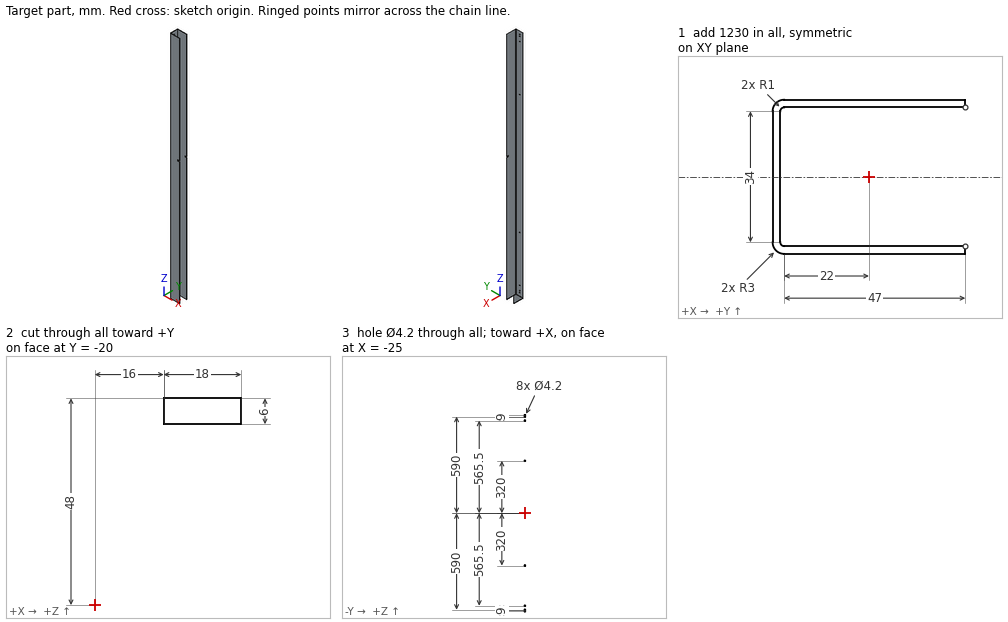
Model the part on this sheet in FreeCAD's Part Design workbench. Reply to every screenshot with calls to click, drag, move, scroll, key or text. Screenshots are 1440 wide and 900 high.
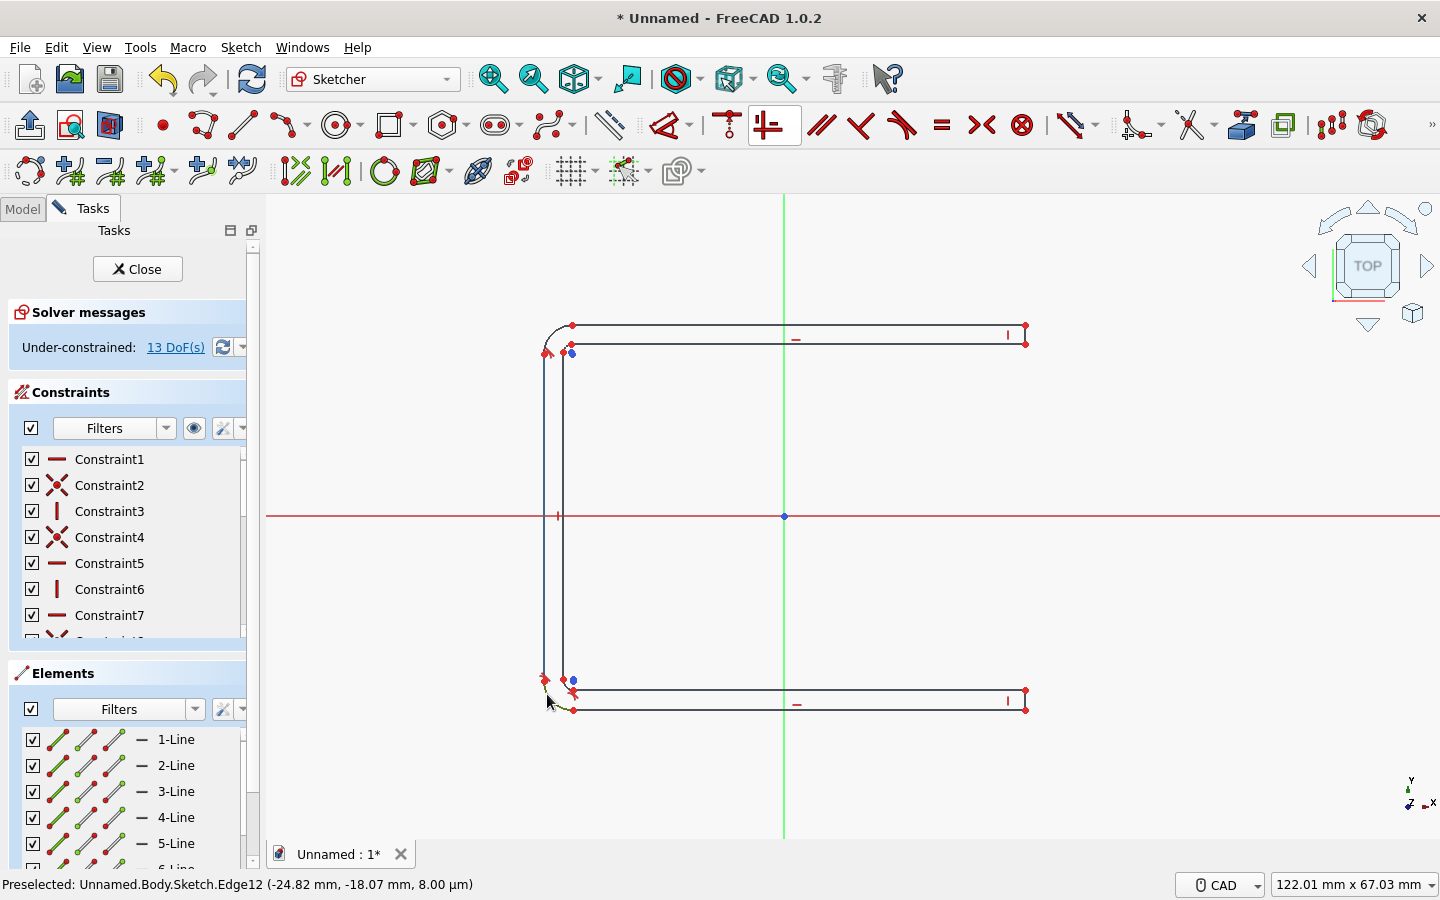
key(t)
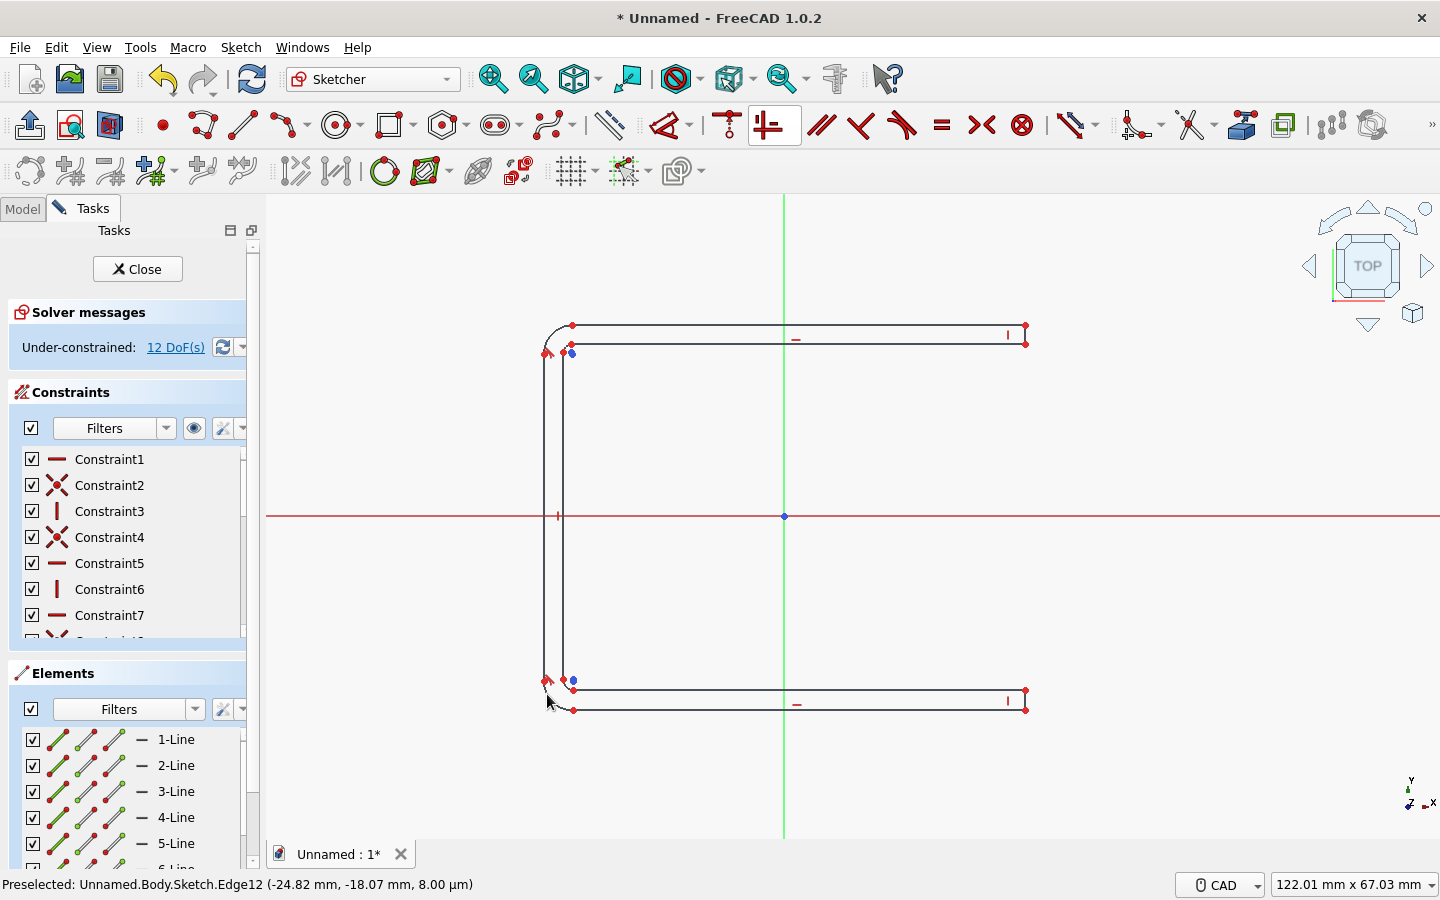
scroll(566, 347, up, 4)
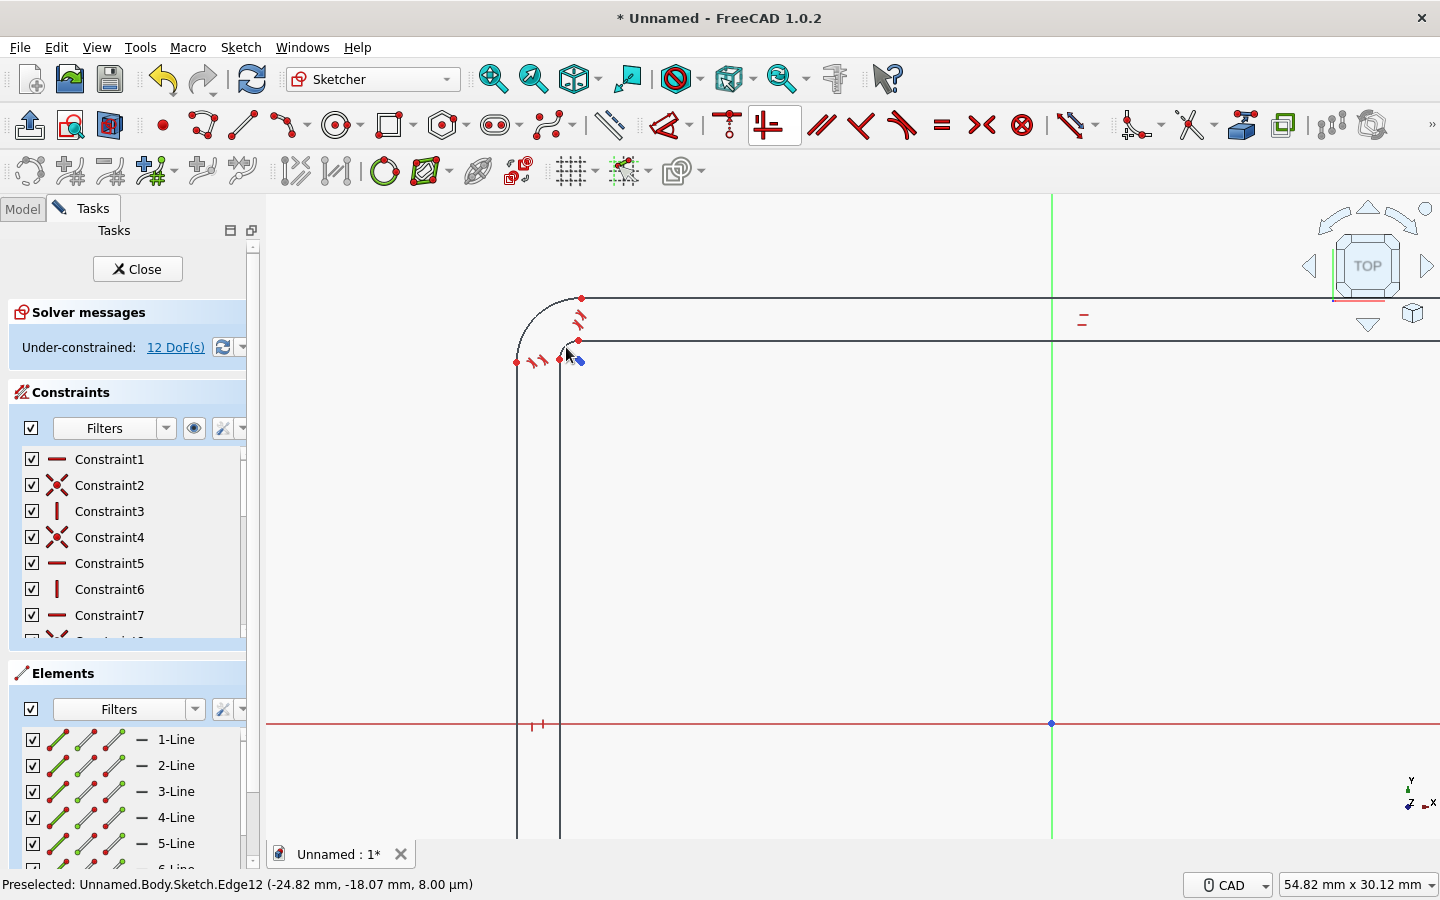
click(565, 346)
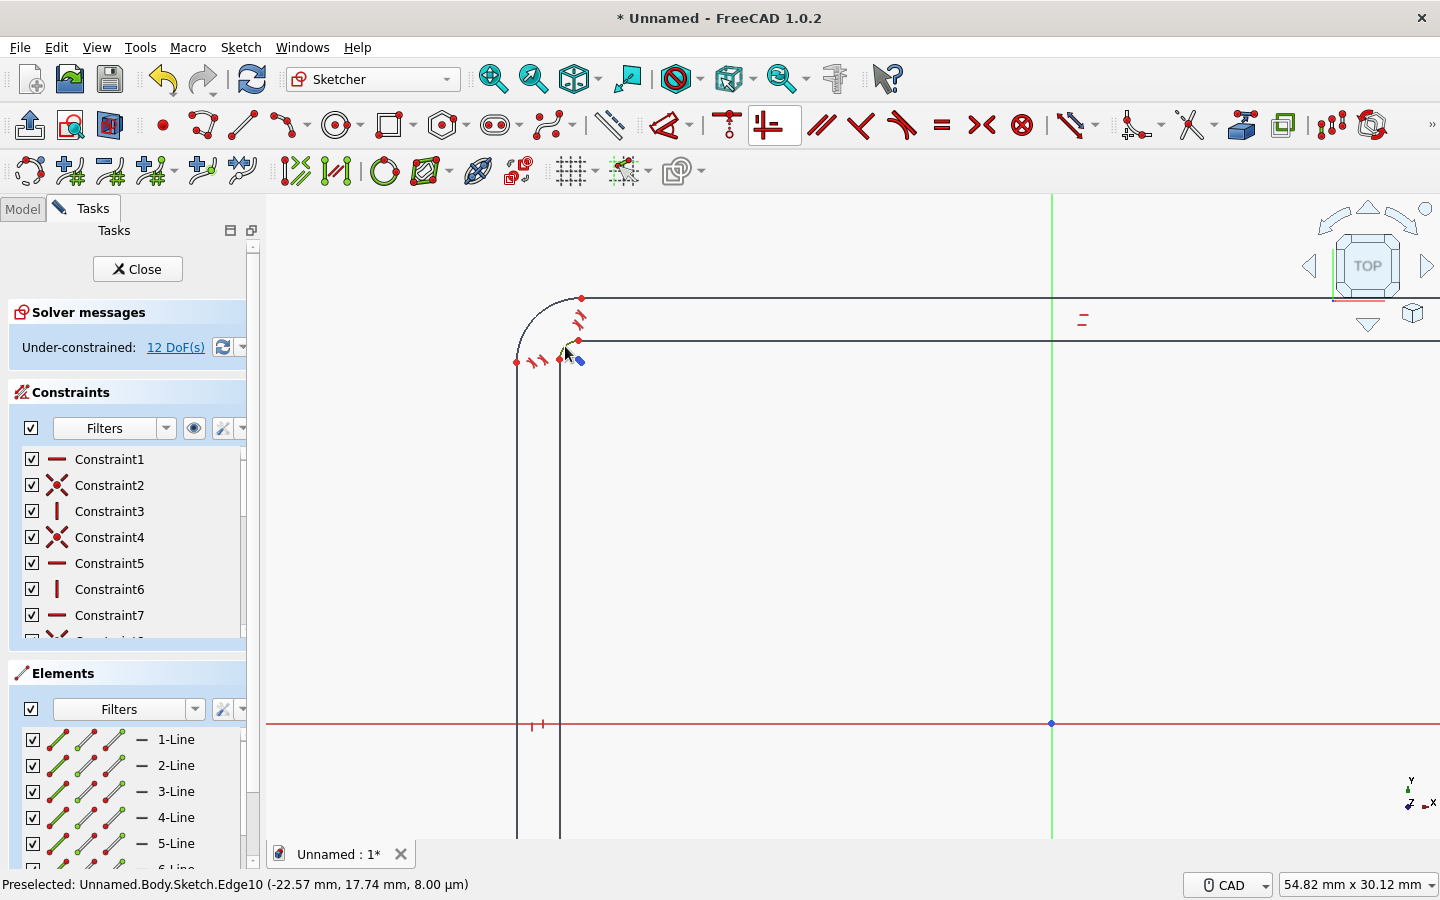
click(552, 305)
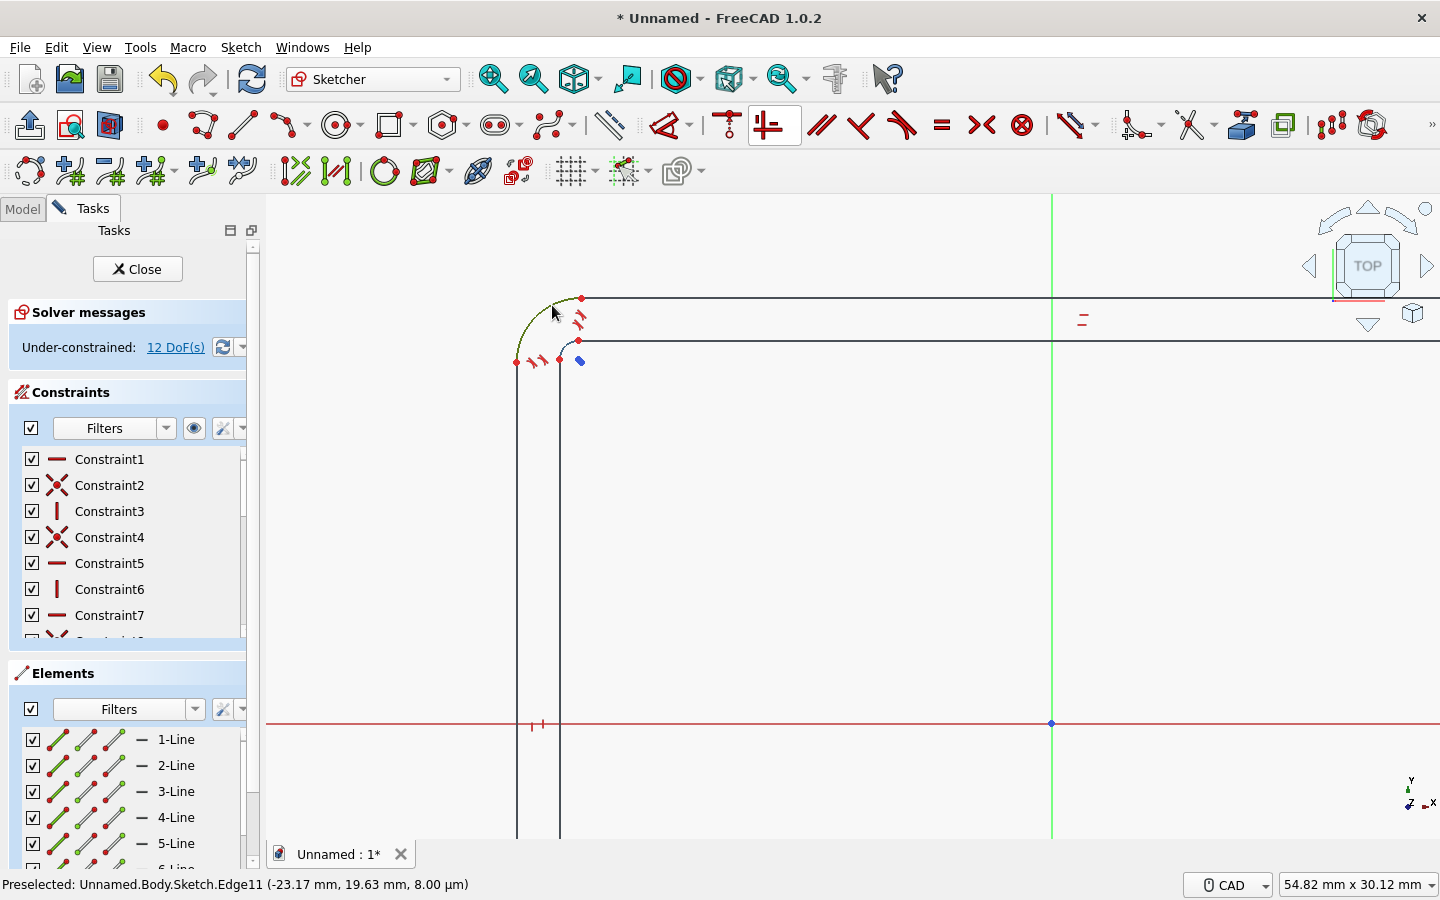
click(728, 126)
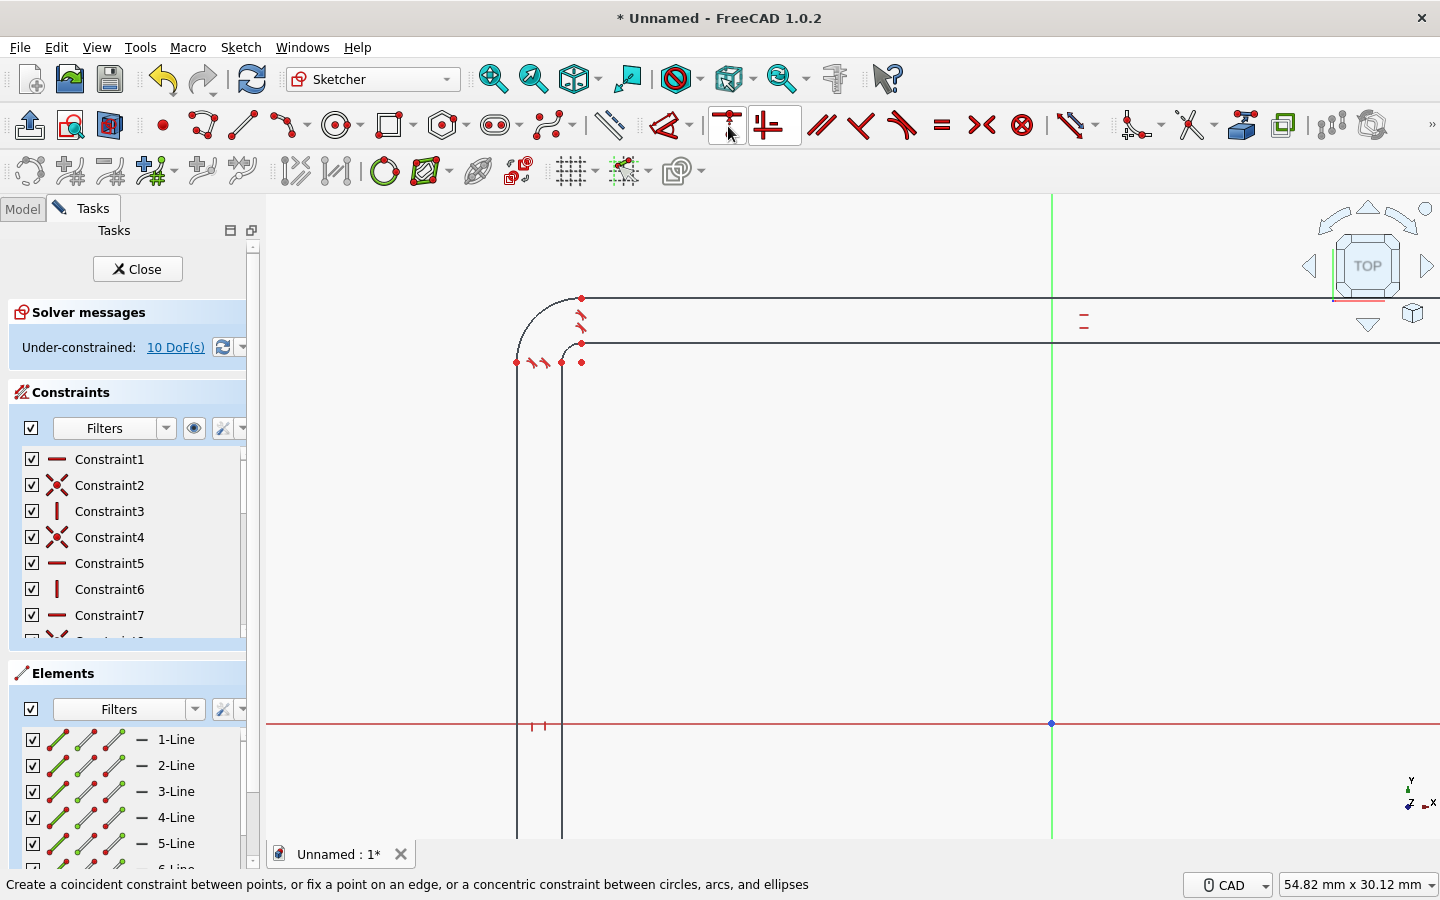
scroll(566, 347, down, 4)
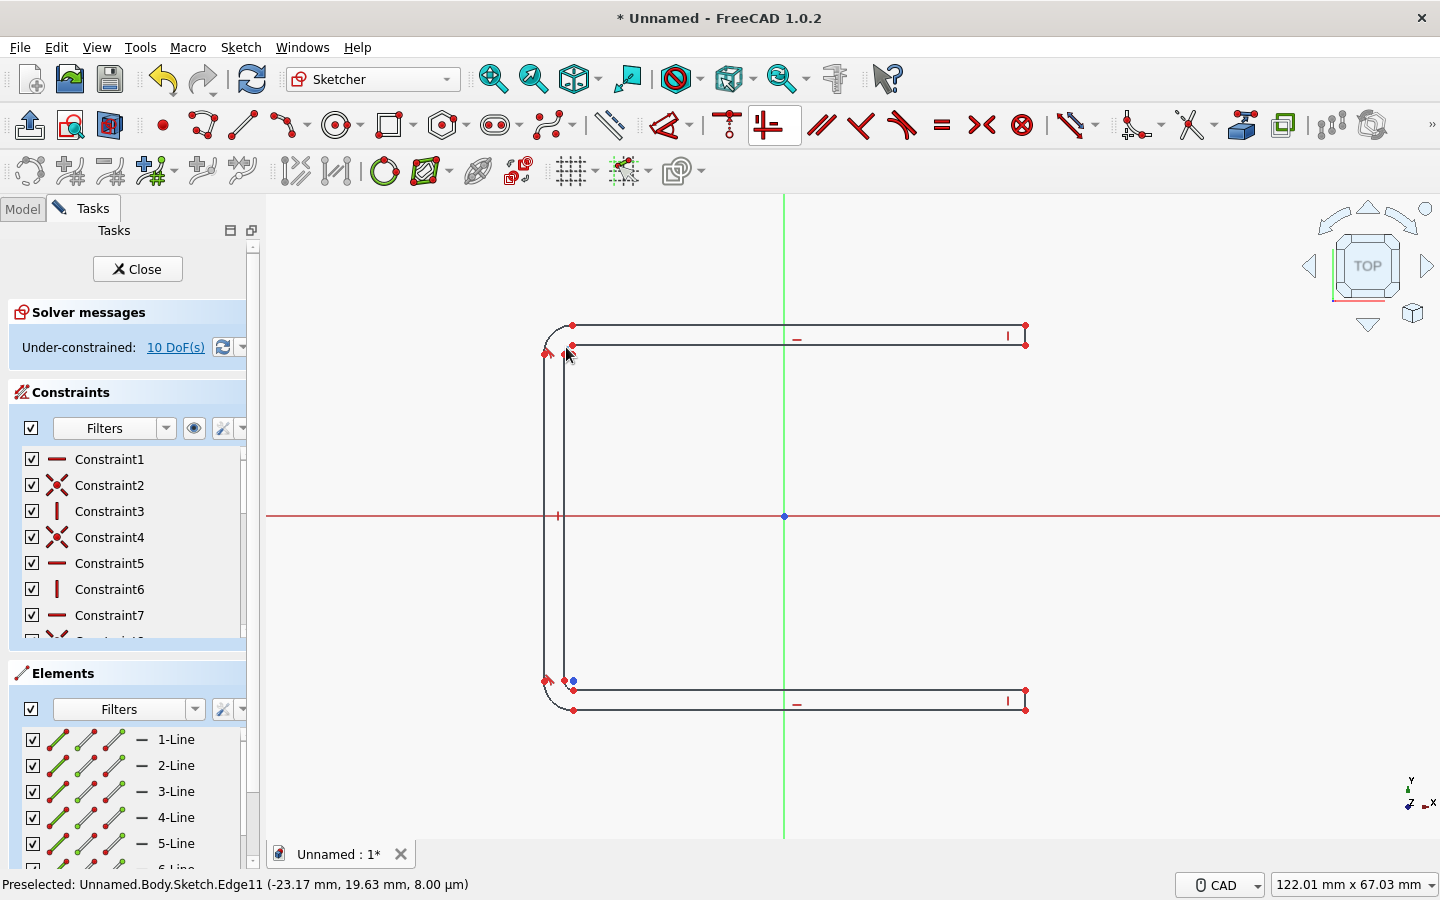
scroll(565, 685, up, 6)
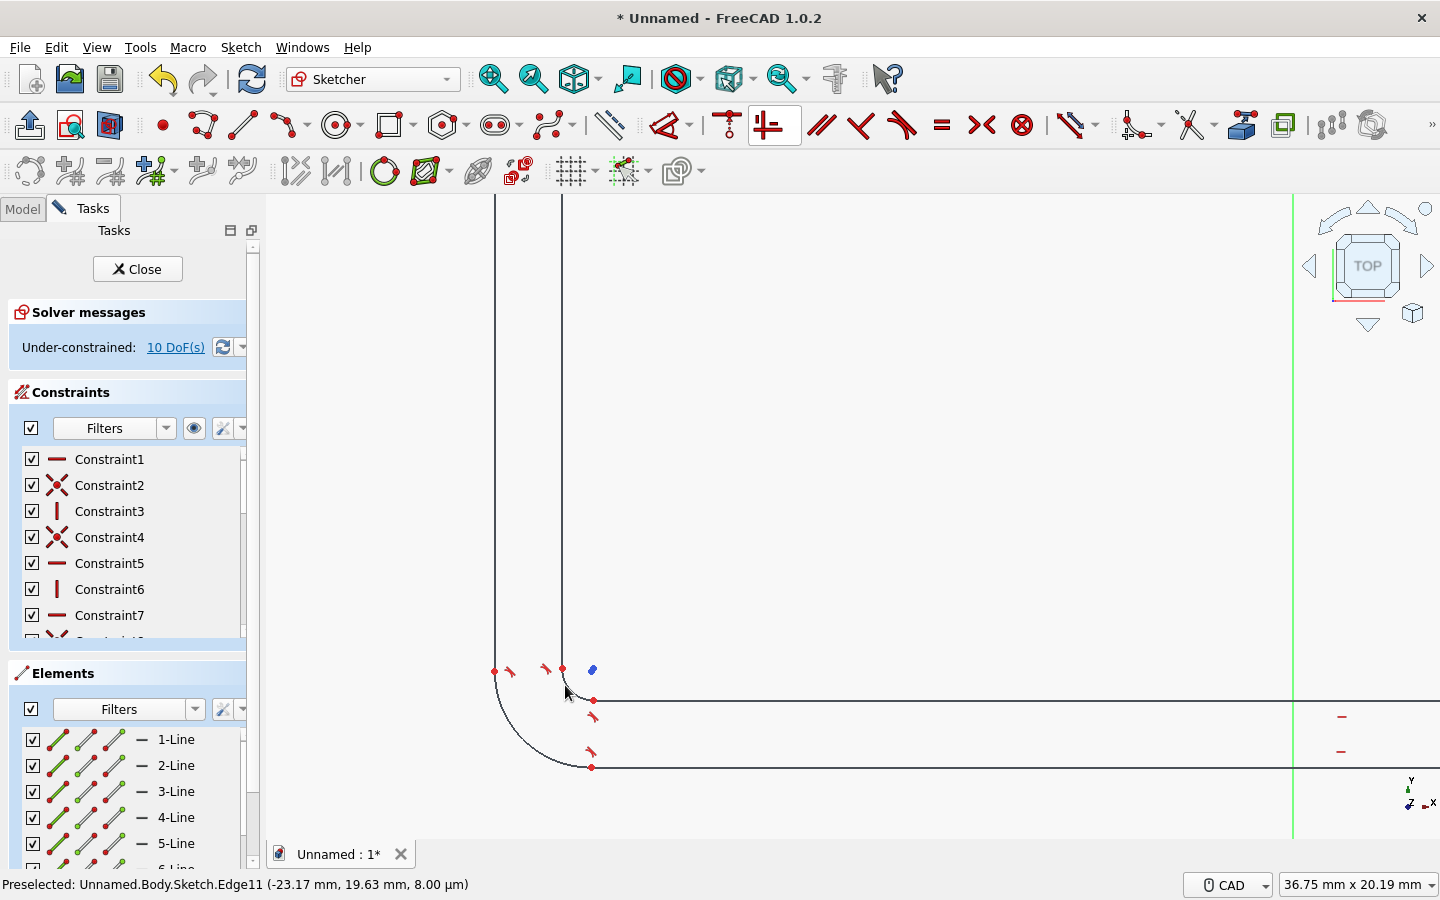
click(566, 683)